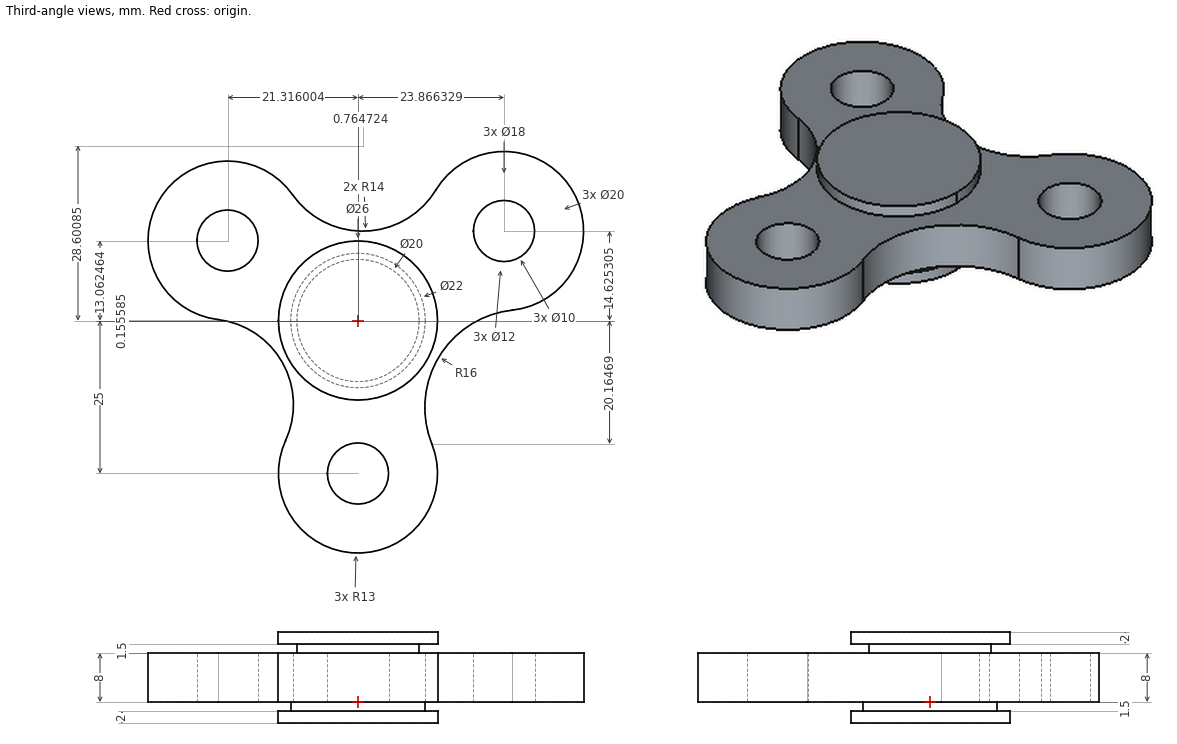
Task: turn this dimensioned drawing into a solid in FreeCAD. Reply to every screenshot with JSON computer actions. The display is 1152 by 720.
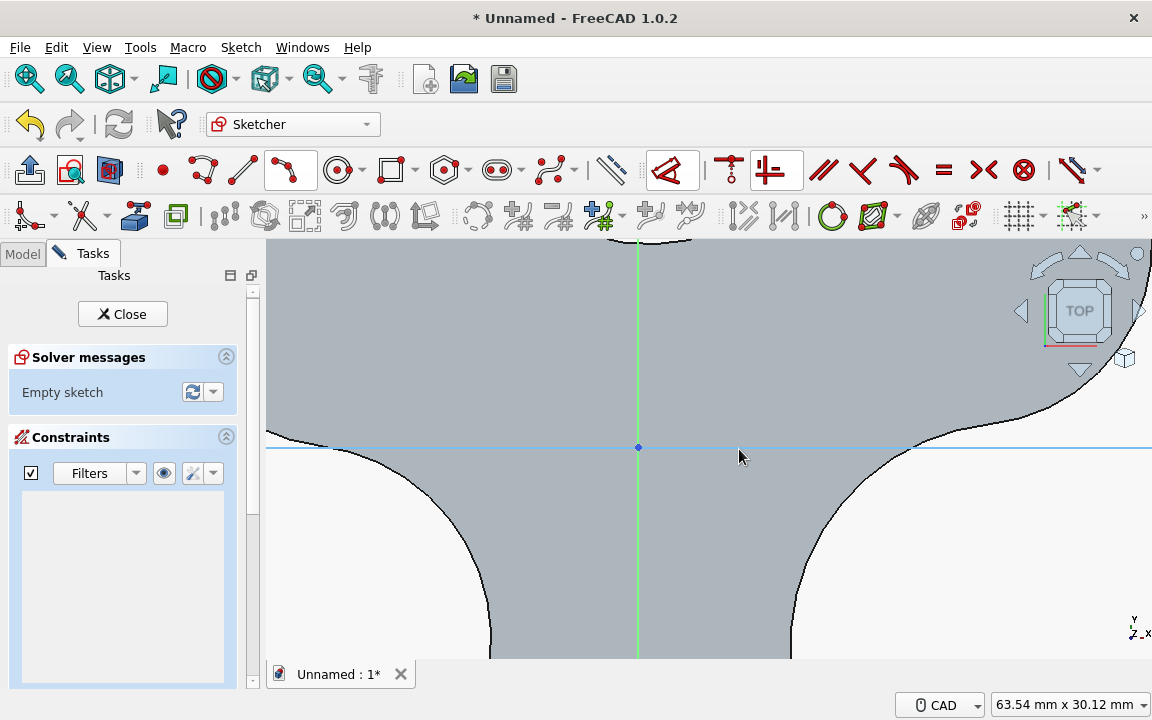
{"action": "left_click", "coordinate": [338, 170]}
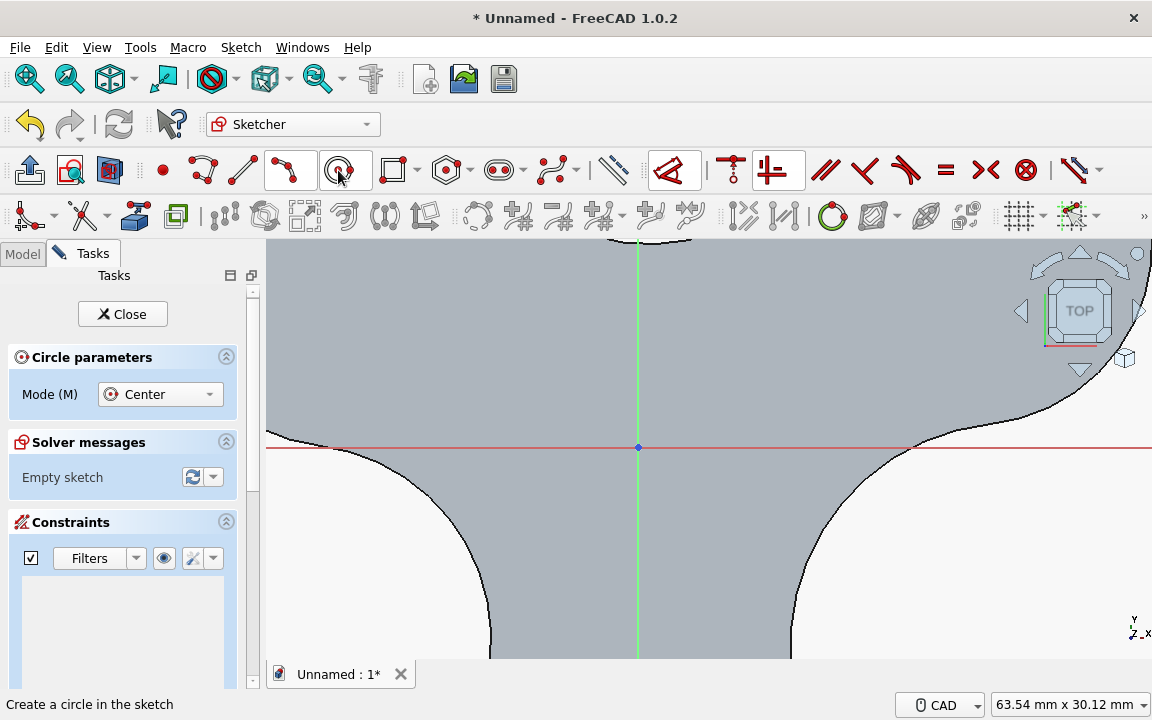
{"action": "left_click", "coordinate": [638, 448]}
{"action": "mouse_move", "coordinate": [737, 349]}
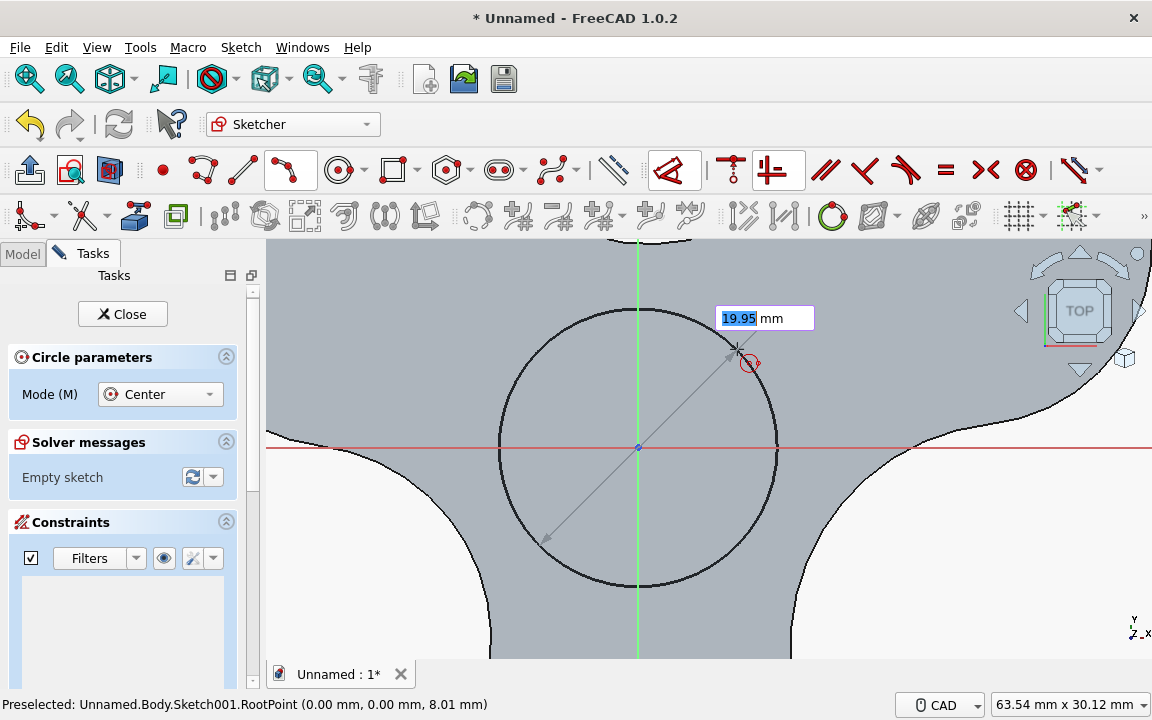
{"action": "type", "text": "20"}
{"action": "key", "text": "Return"}
{"action": "key", "text": "Escape"}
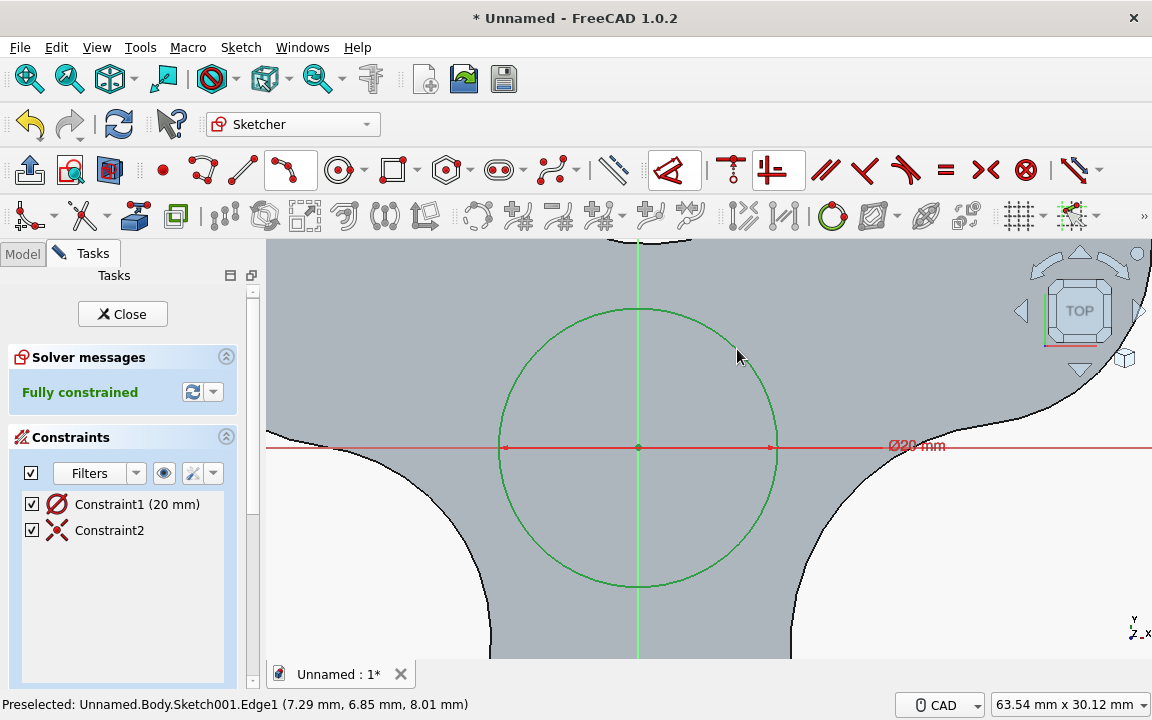
{"action": "left_click", "coordinate": [123, 314]}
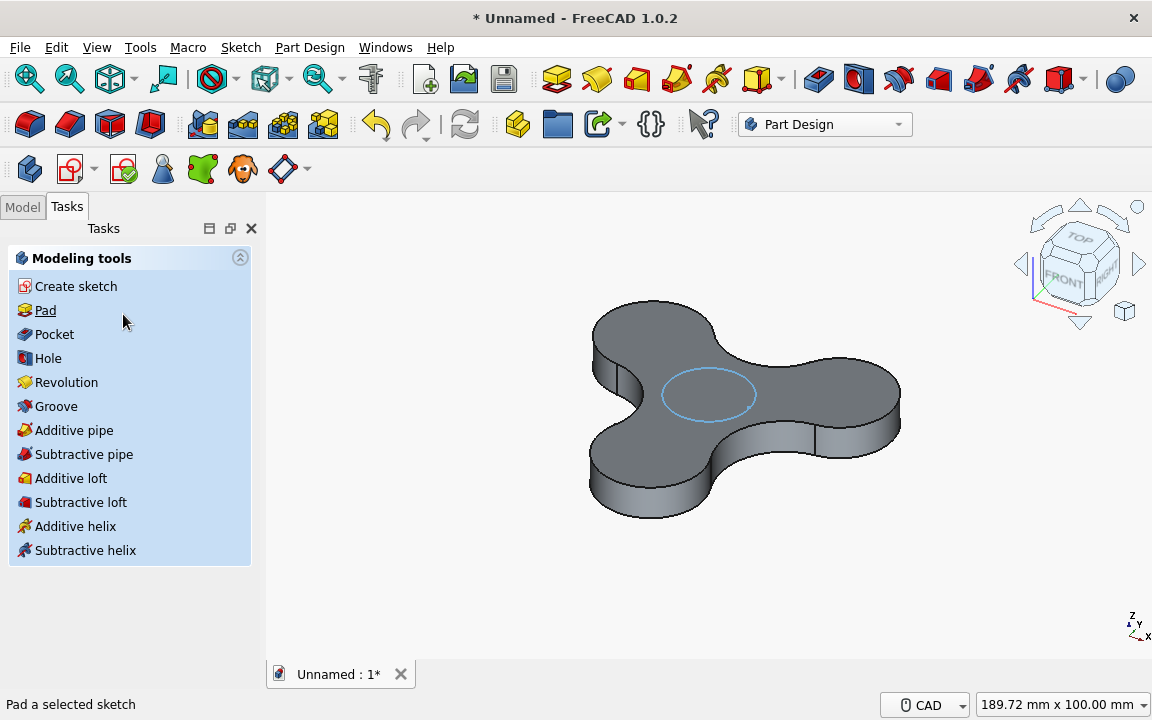
{"action": "left_click", "coordinate": [558, 80]}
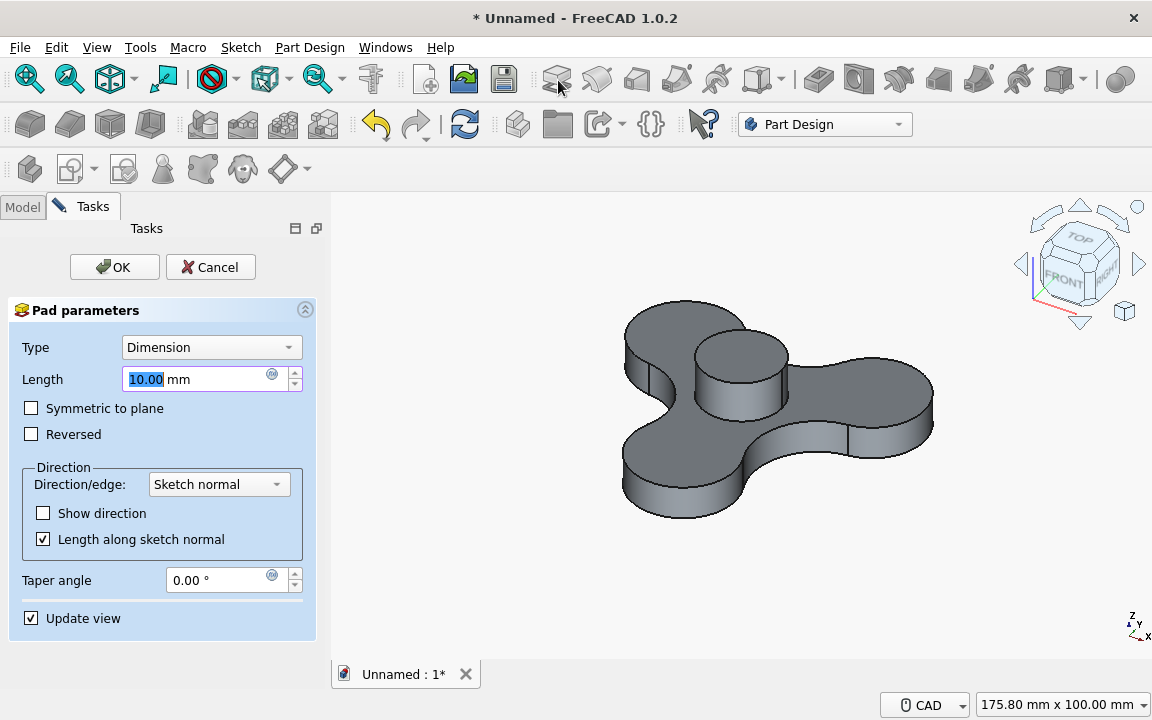
{"action": "type", "text": "1.5"}
{"action": "key", "text": "Tab"}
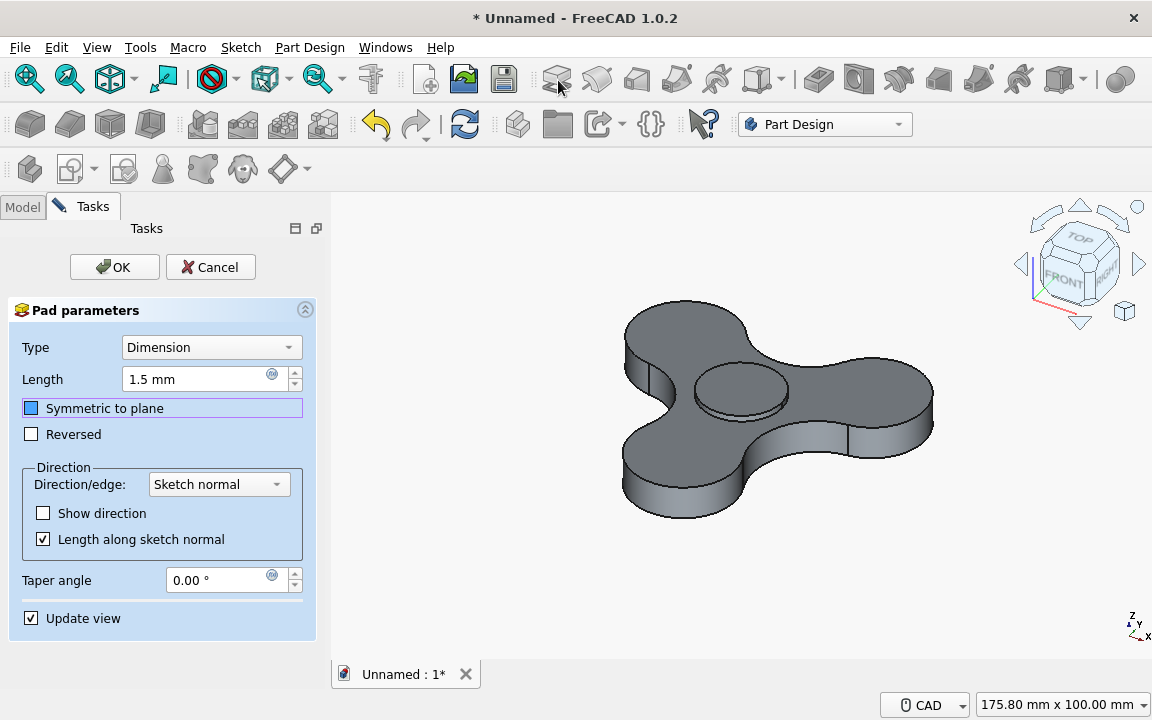
{"action": "left_click", "coordinate": [115, 267]}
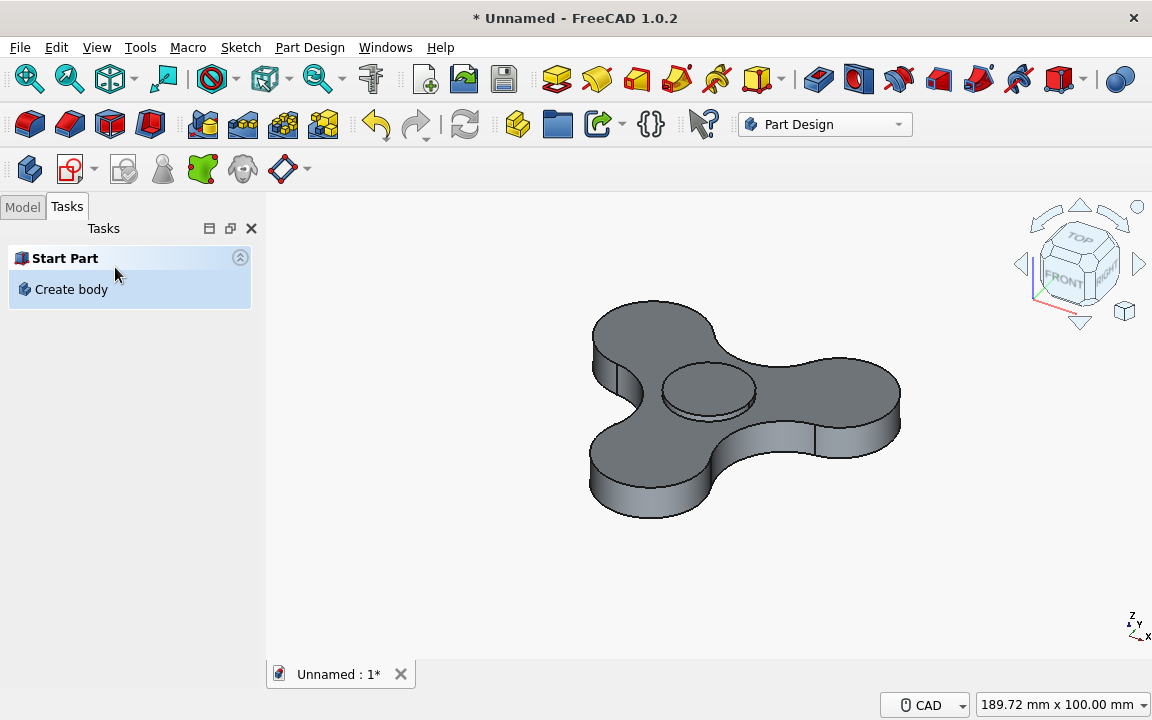
{"action": "key", "text": "5"}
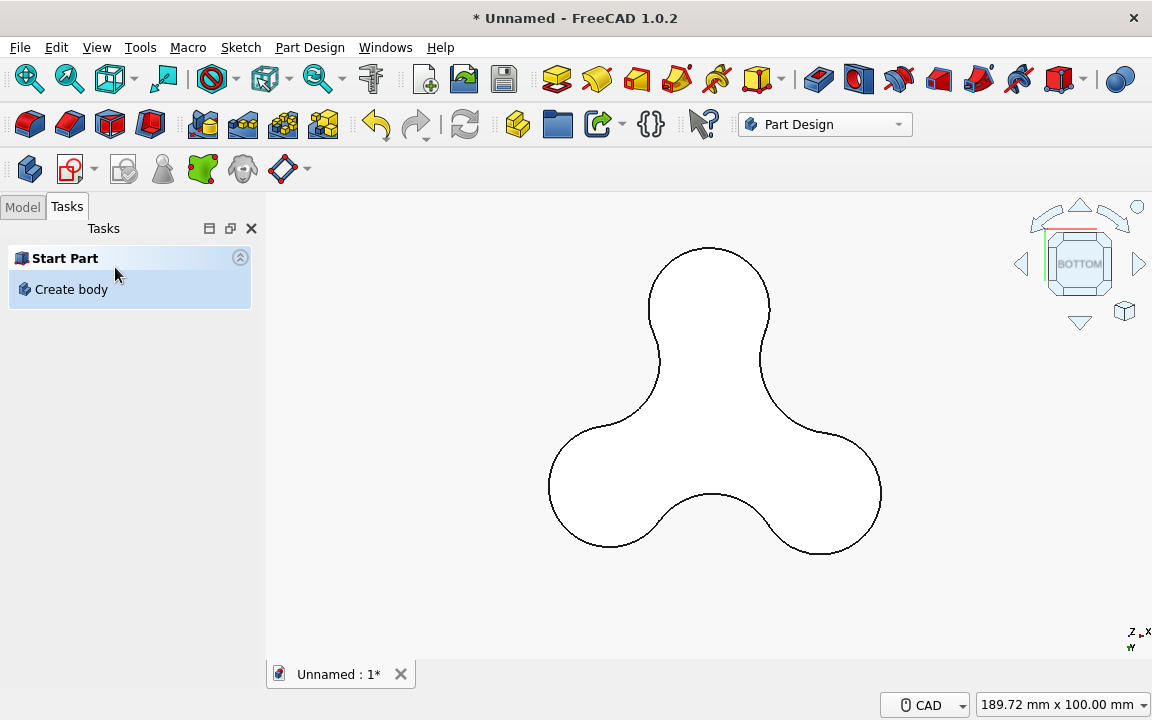
{"action": "left_click", "coordinate": [810, 488]}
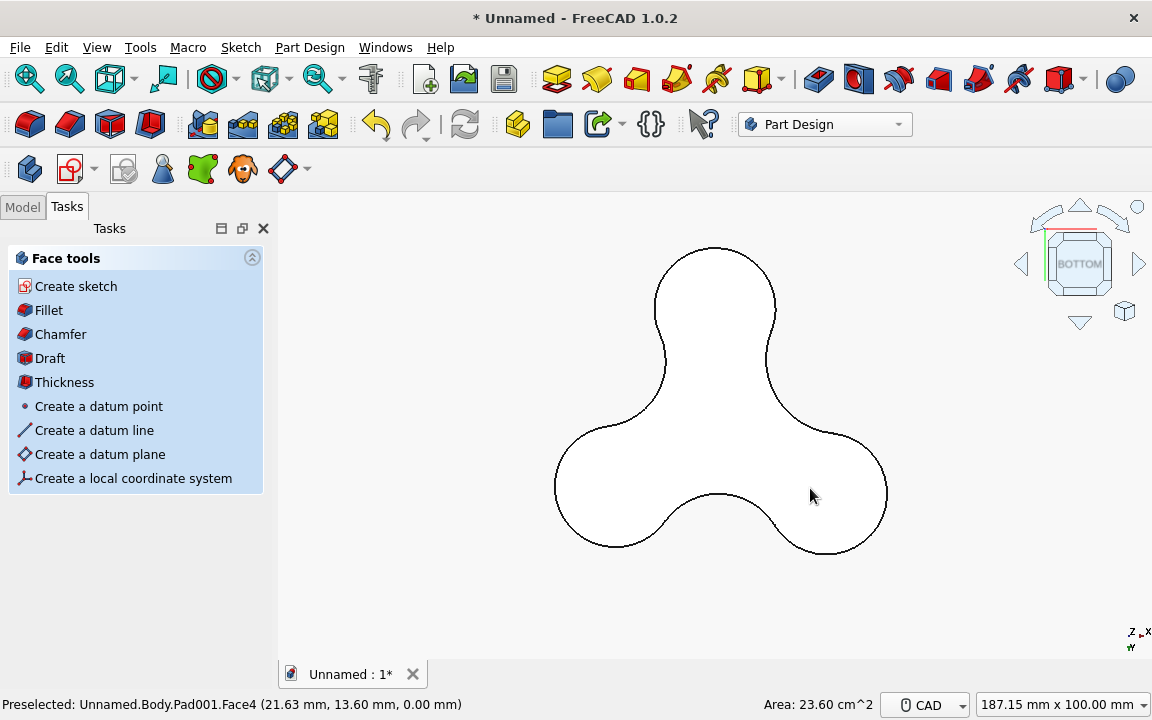
{"action": "left_click", "coordinate": [70, 170]}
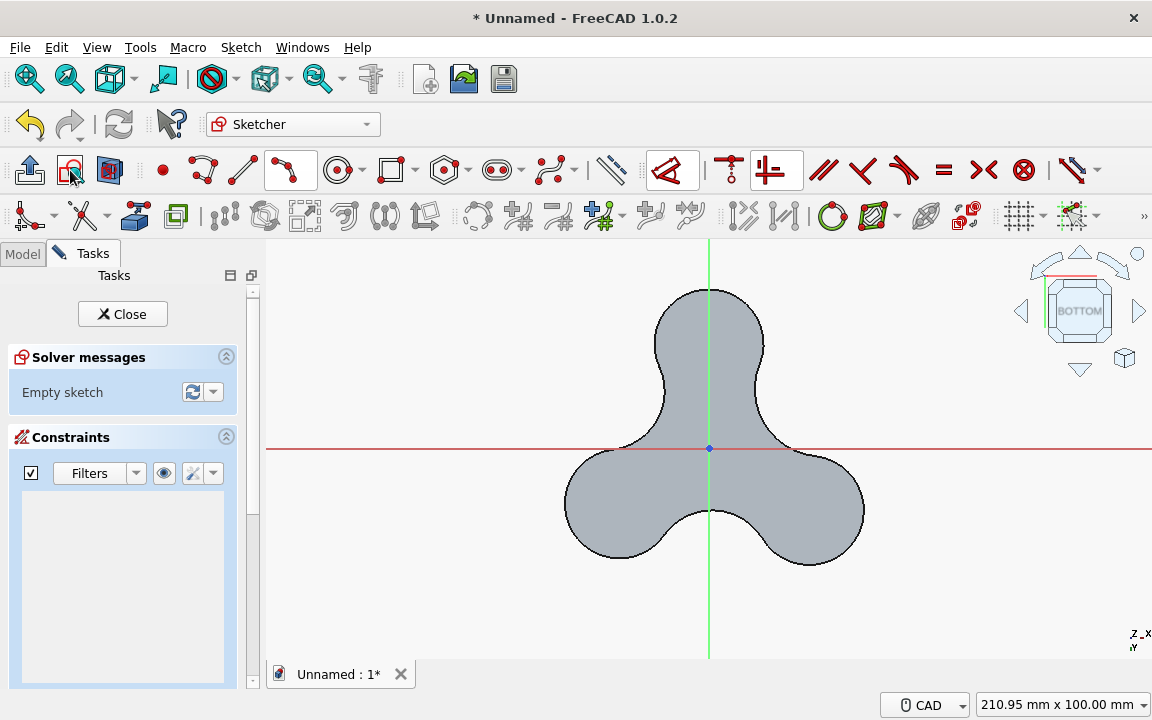
{"action": "scroll", "coordinate": [749, 449], "scroll_direction": "up", "scroll_amount": 5}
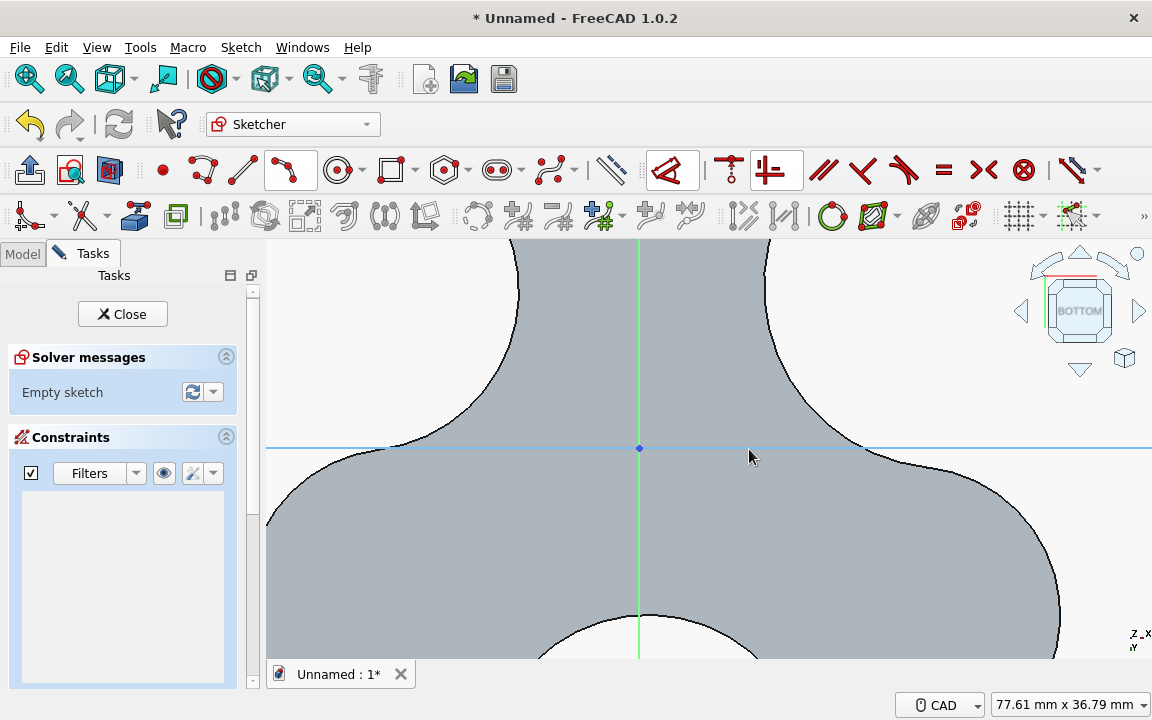
{"action": "left_click", "coordinate": [338, 170]}